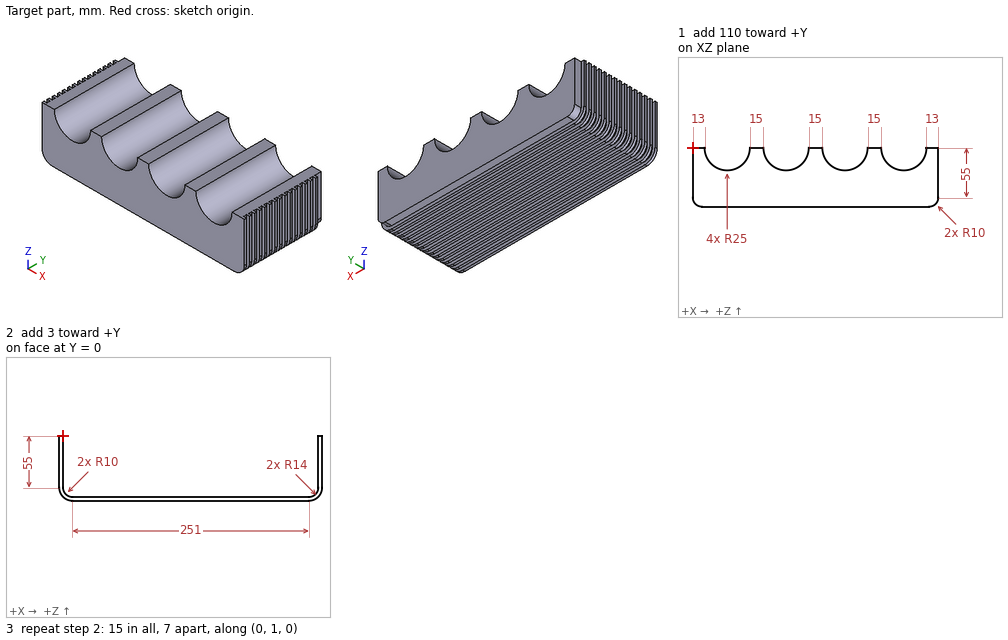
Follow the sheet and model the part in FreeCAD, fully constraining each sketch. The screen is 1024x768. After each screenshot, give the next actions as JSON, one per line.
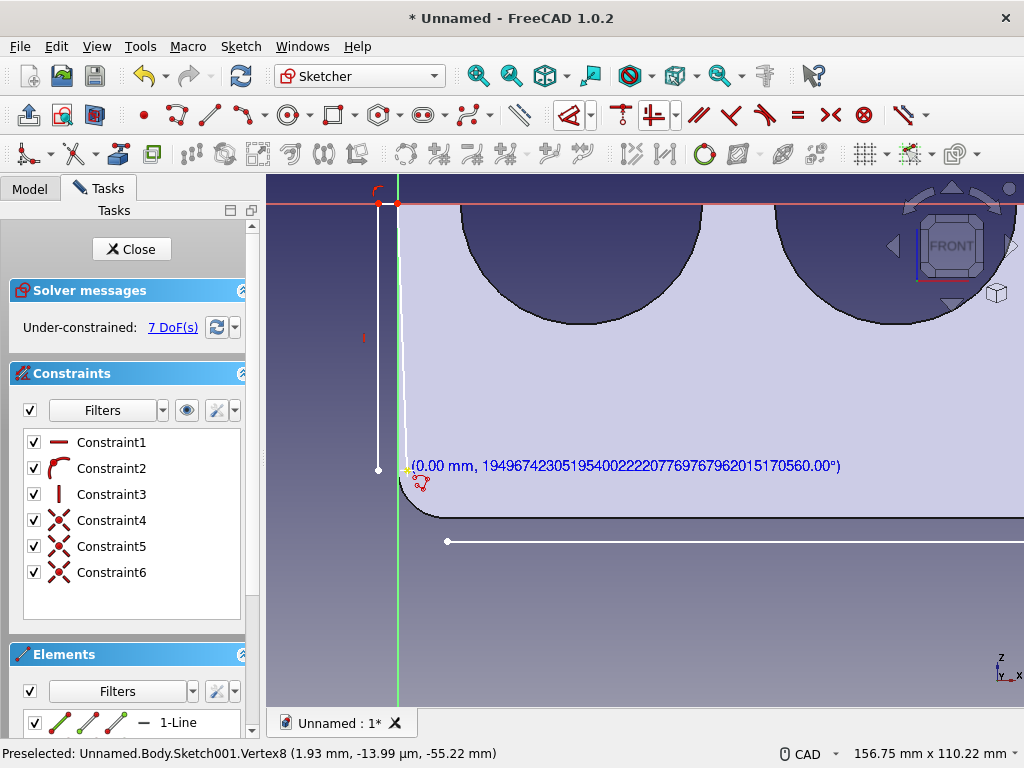
{"action": "left_click", "coordinate": [210, 116]}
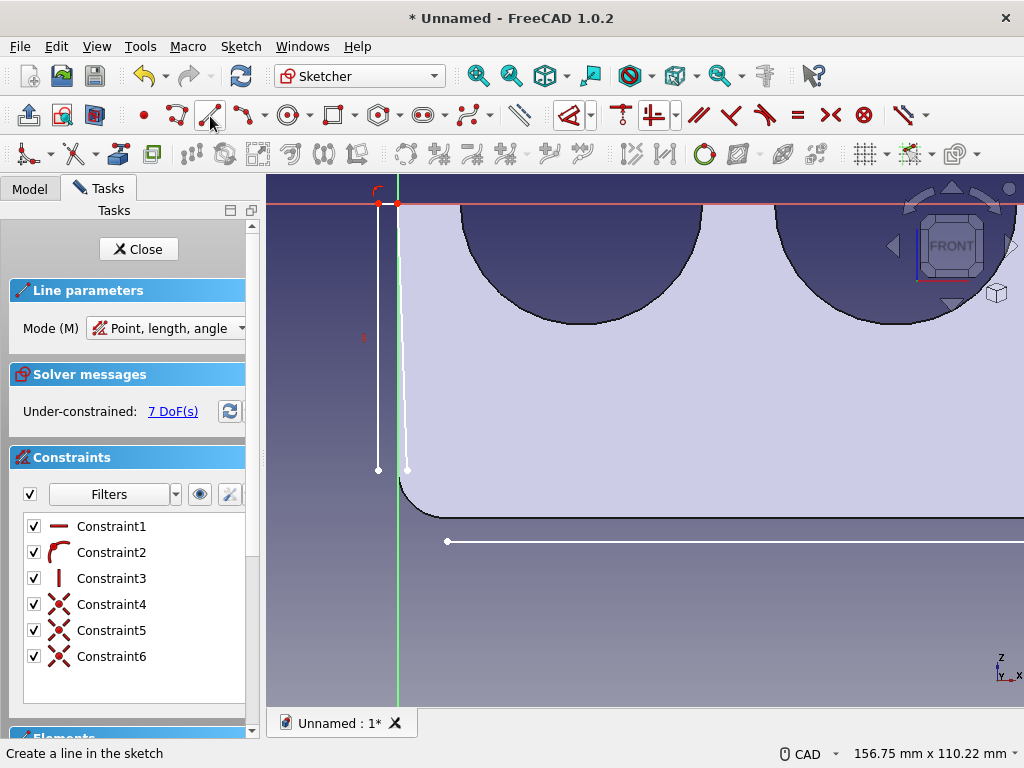
{"action": "left_click", "coordinate": [446, 518]}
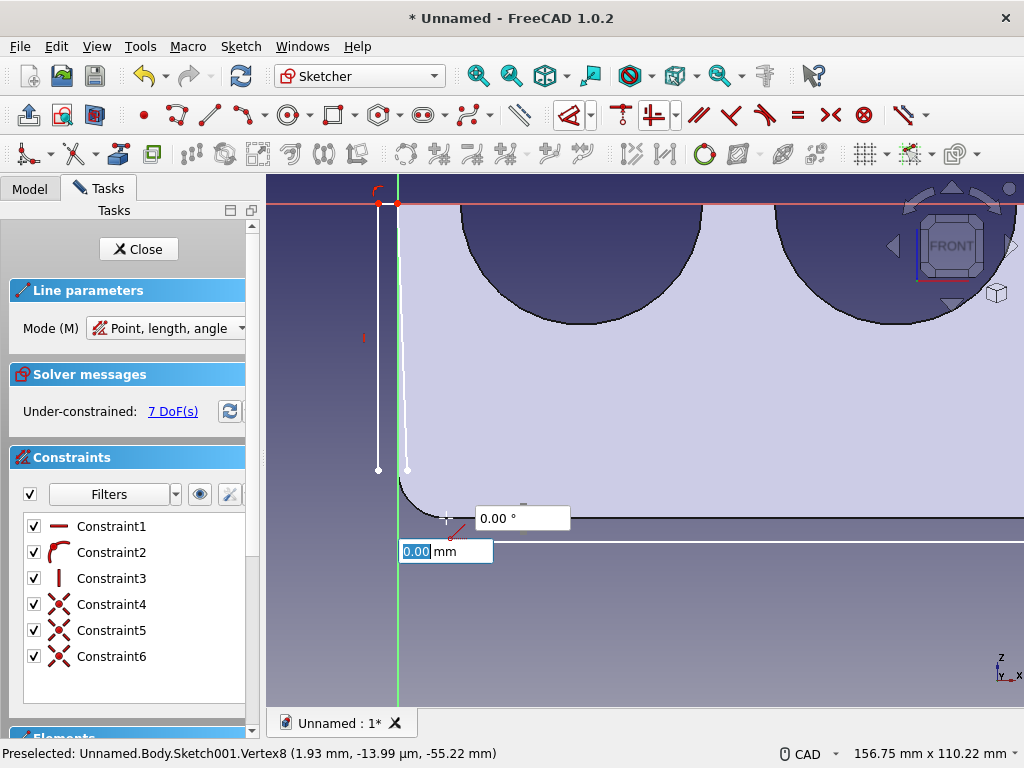
{"action": "scroll", "coordinate": [371, 471], "scroll_direction": "down", "scroll_amount": 6}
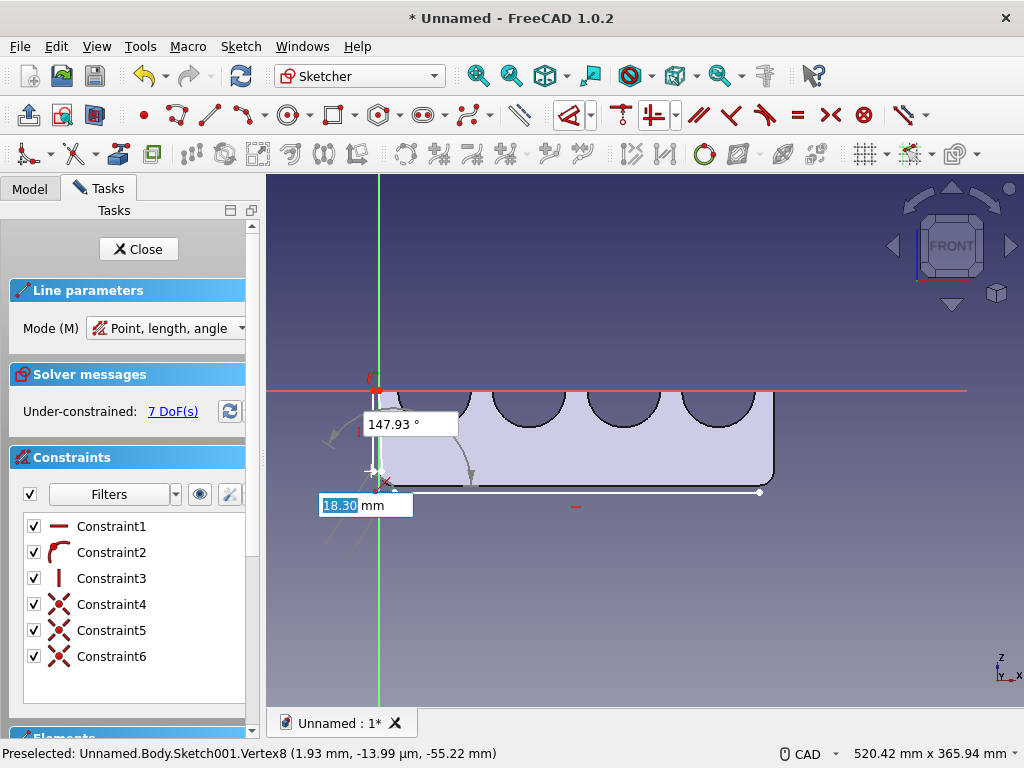
{"action": "scroll", "coordinate": [759, 486], "scroll_direction": "up", "scroll_amount": 6}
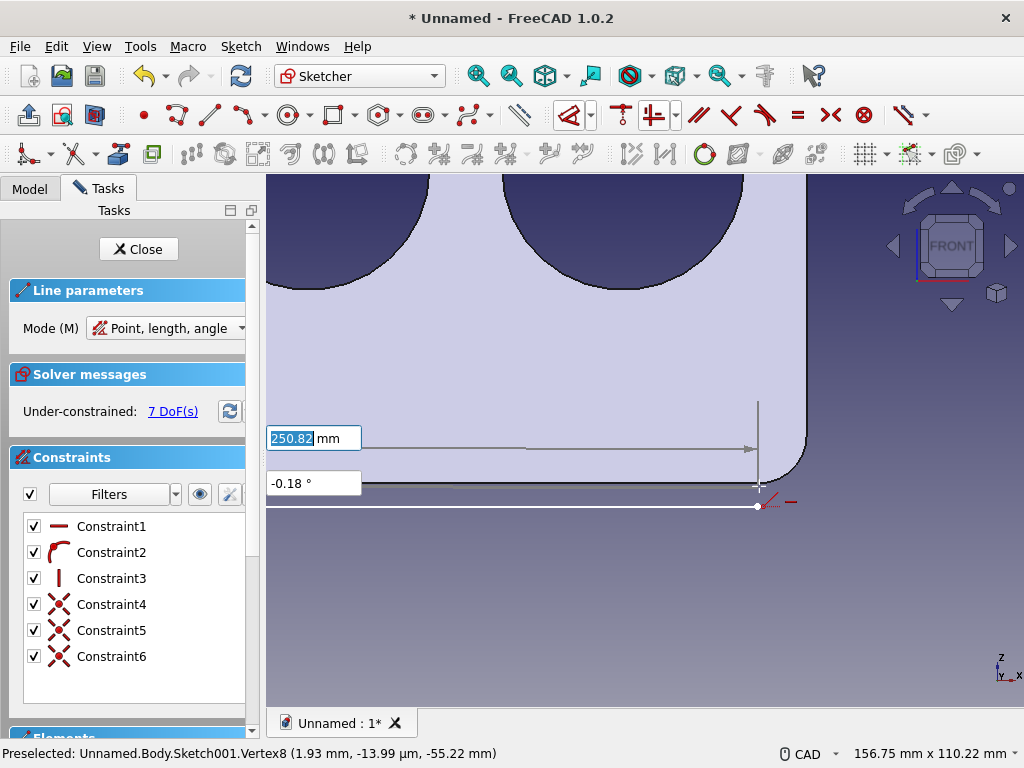
{"action": "left_click", "coordinate": [758, 483]}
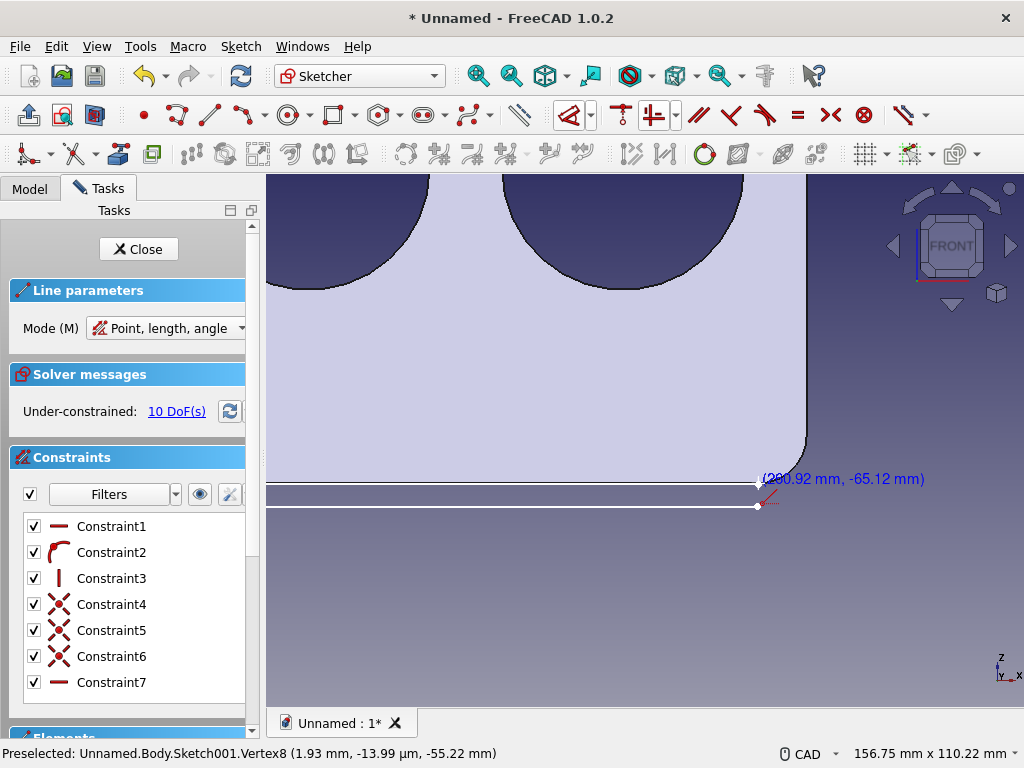
{"action": "left_click", "coordinate": [177, 116]}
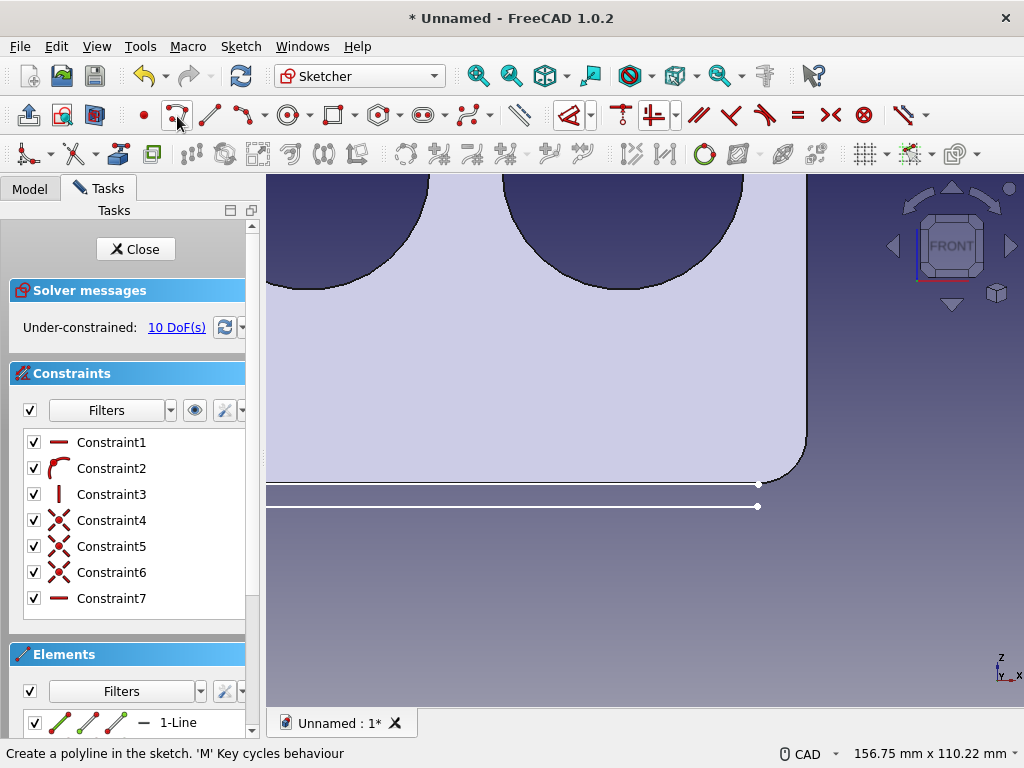
{"action": "left_click", "coordinate": [807, 435]}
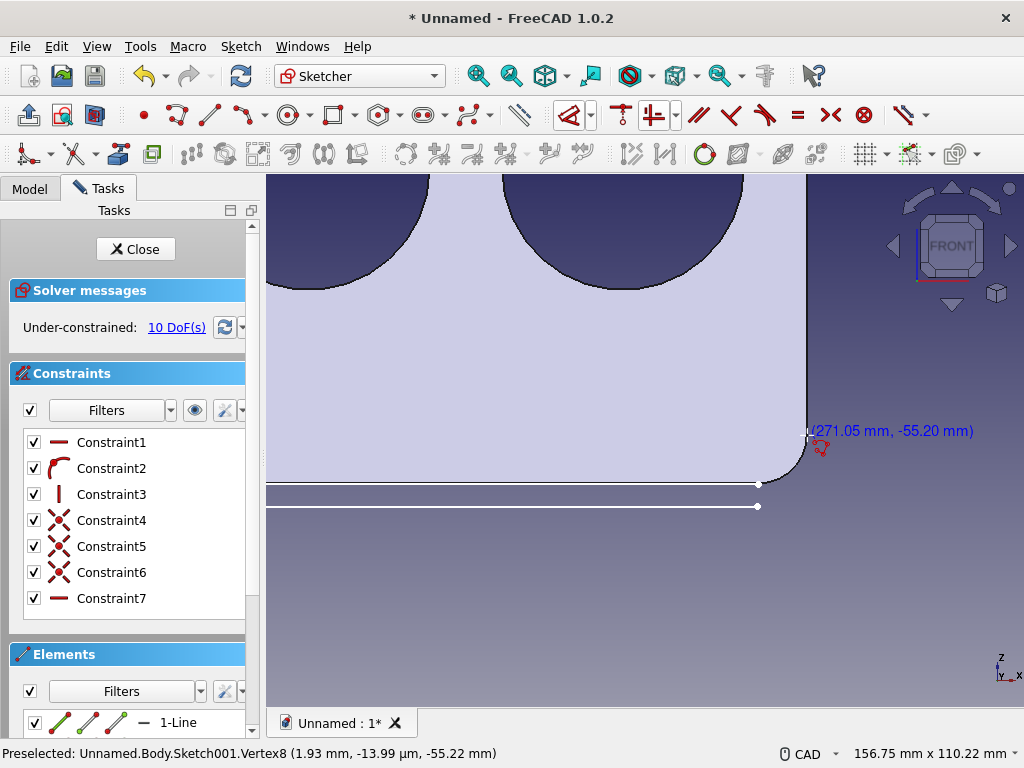
{"action": "scroll", "coordinate": [760, 486], "scroll_direction": "down", "scroll_amount": 6}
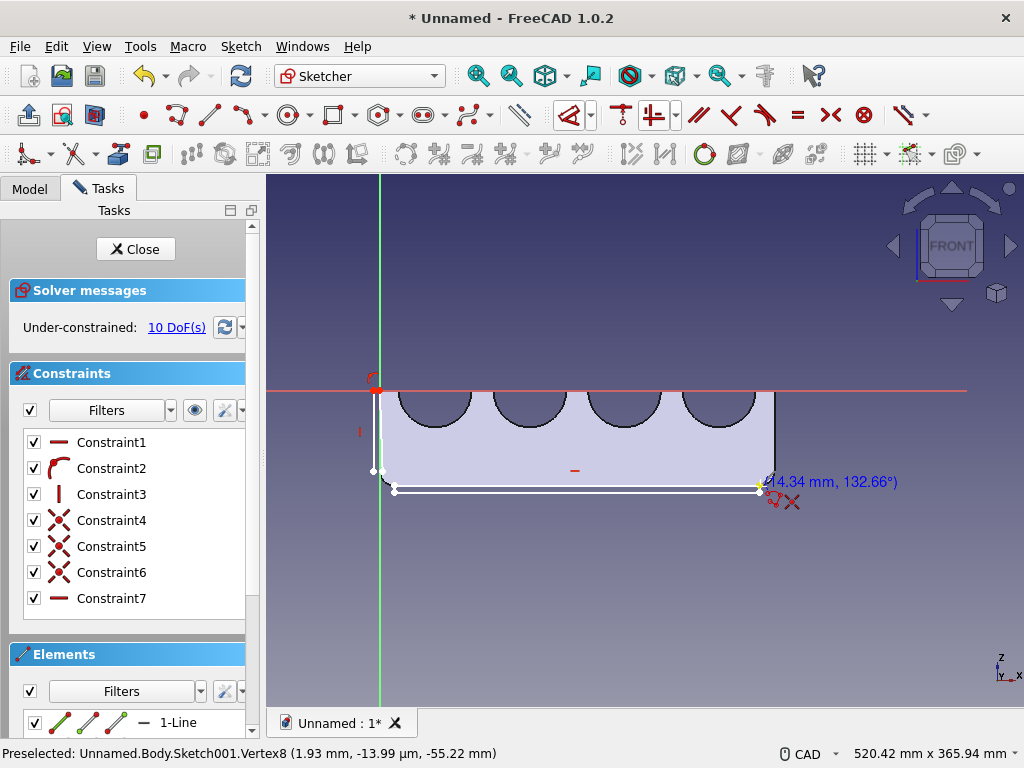
{"action": "left_click", "coordinate": [775, 391]}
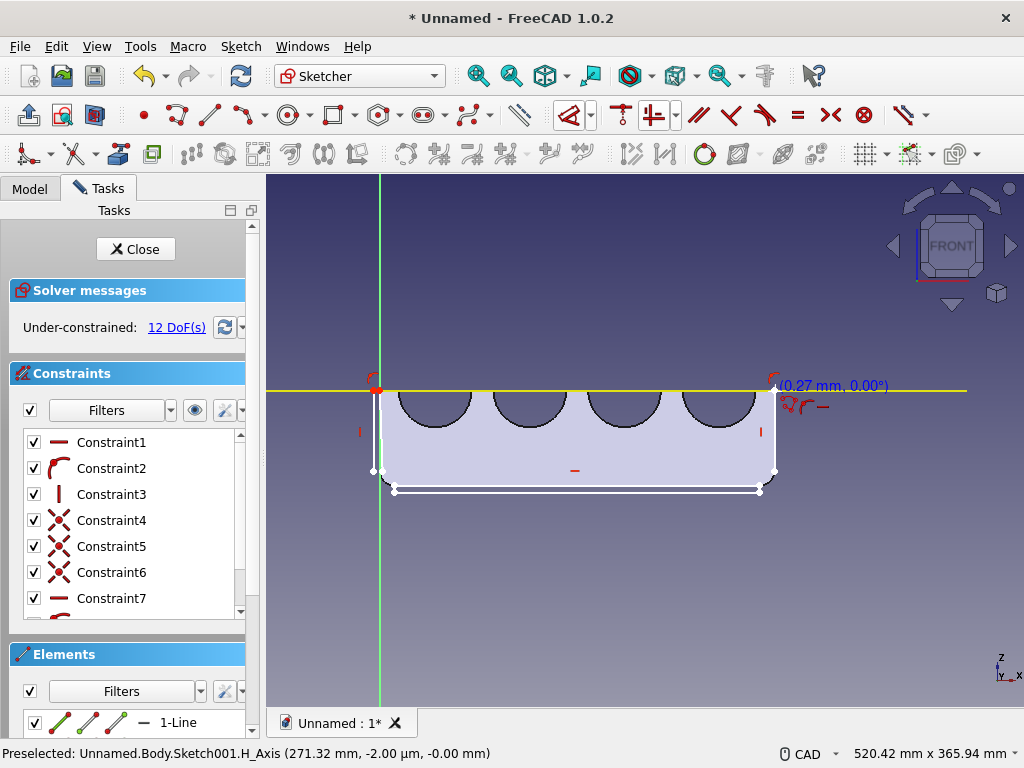
{"action": "scroll", "coordinate": [780, 391], "scroll_direction": "up", "scroll_amount": 6}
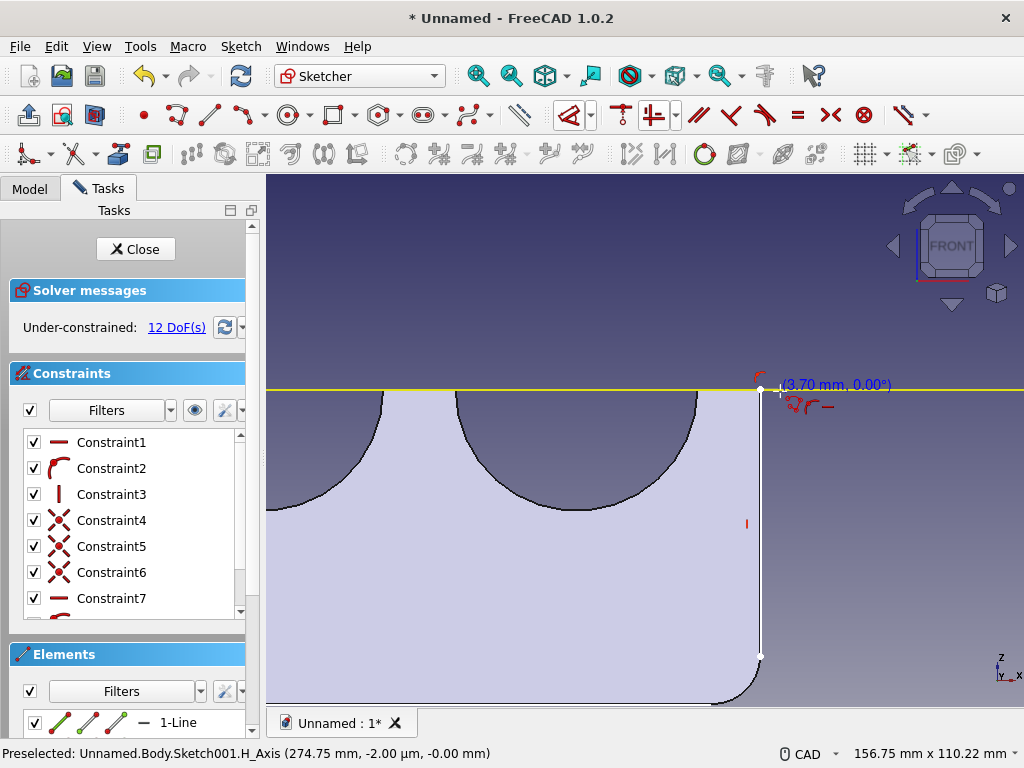
{"action": "left_click", "coordinate": [780, 399]}
{"action": "left_click", "coordinate": [780, 656]}
{"action": "right_click", "coordinate": [780, 656]}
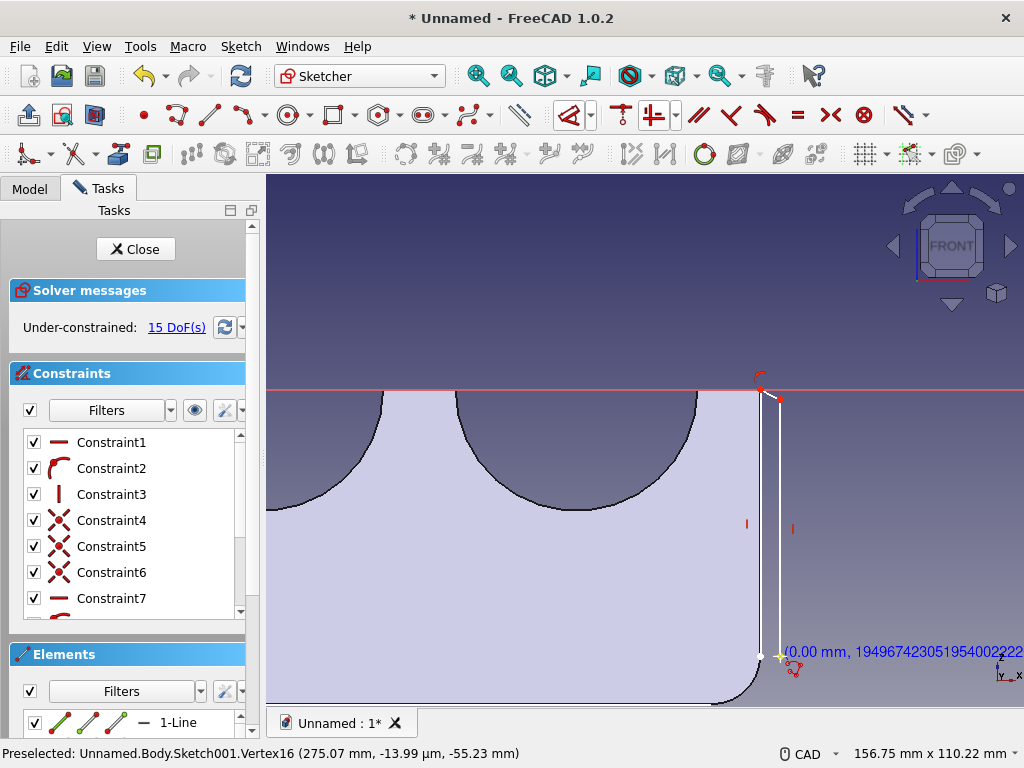
{"action": "left_click", "coordinate": [242, 116]}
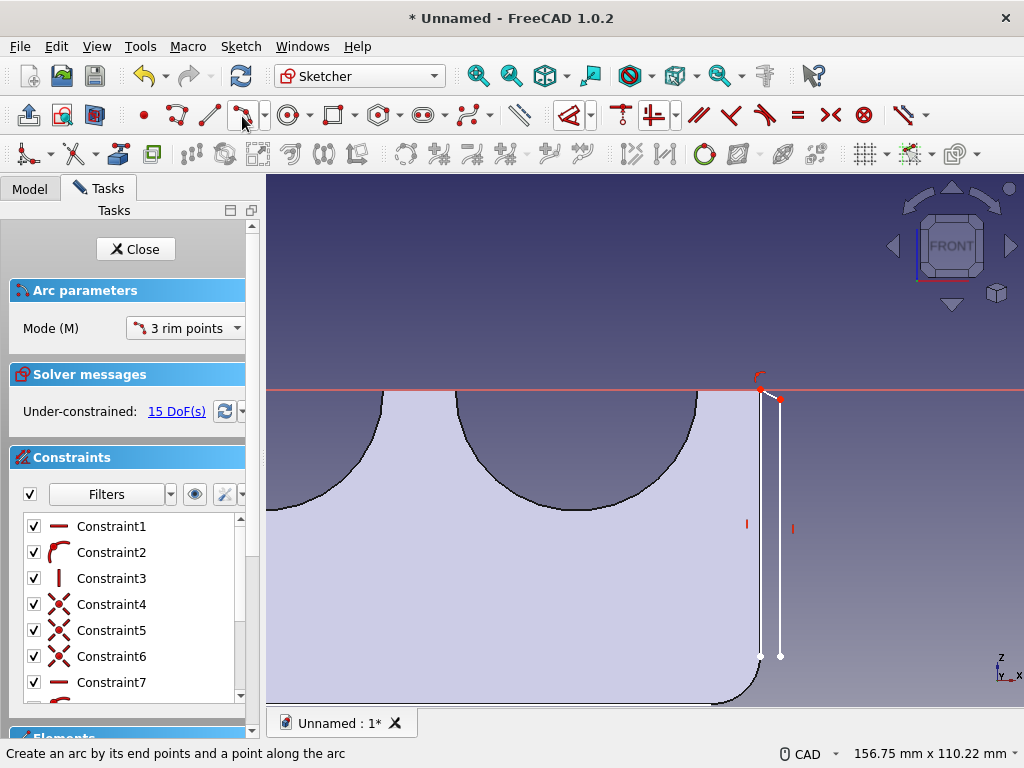
{"action": "scroll", "coordinate": [780, 390], "scroll_direction": "down", "scroll_amount": 6}